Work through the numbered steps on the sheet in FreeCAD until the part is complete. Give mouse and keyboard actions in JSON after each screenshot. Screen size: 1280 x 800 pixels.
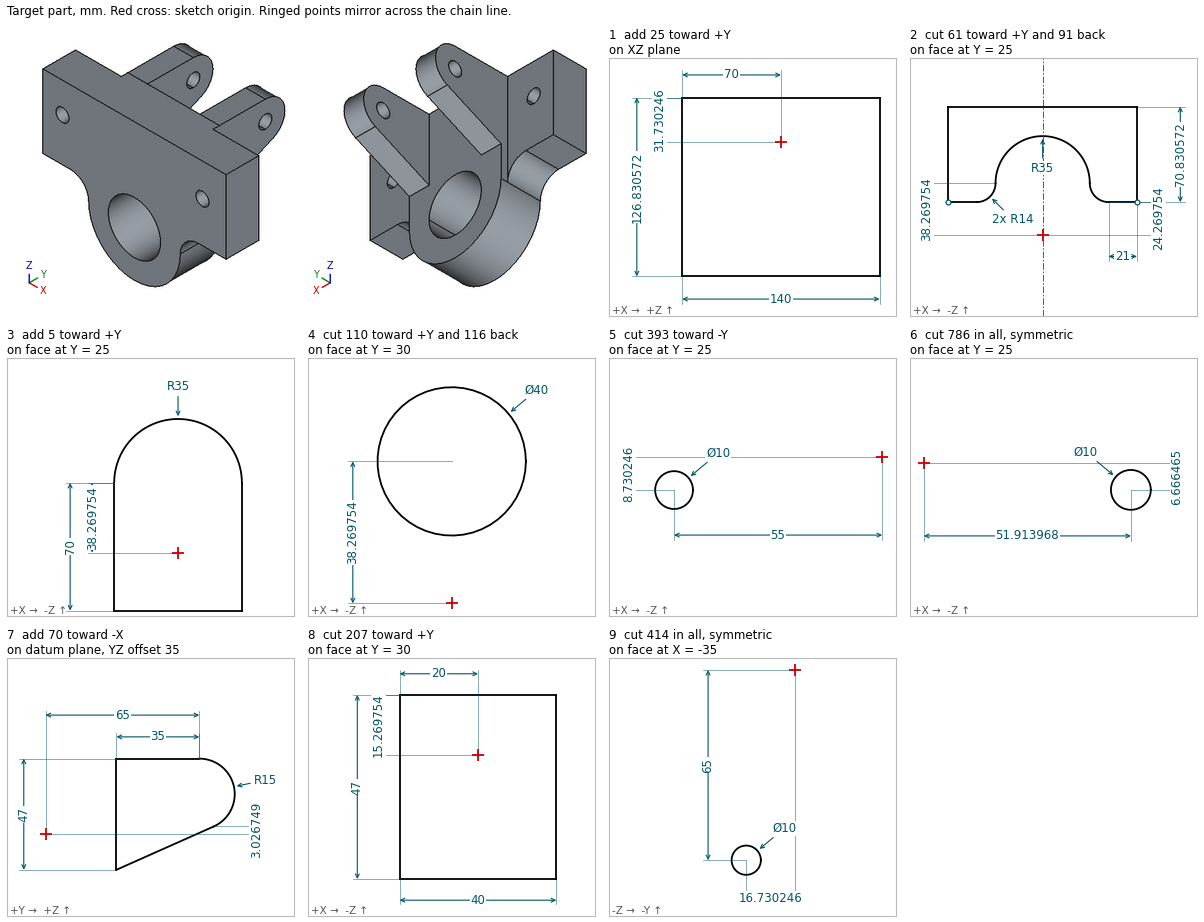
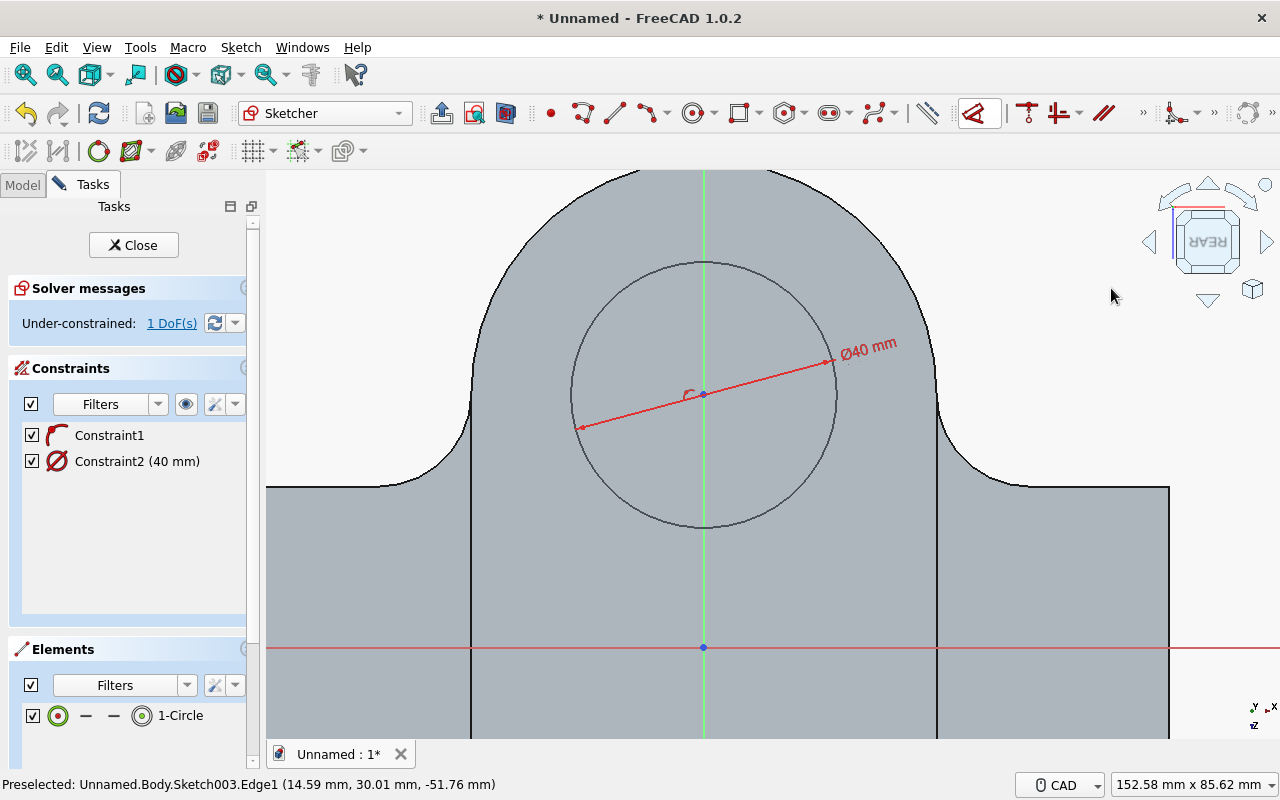
{"action": "left_click", "coordinate": [704, 395]}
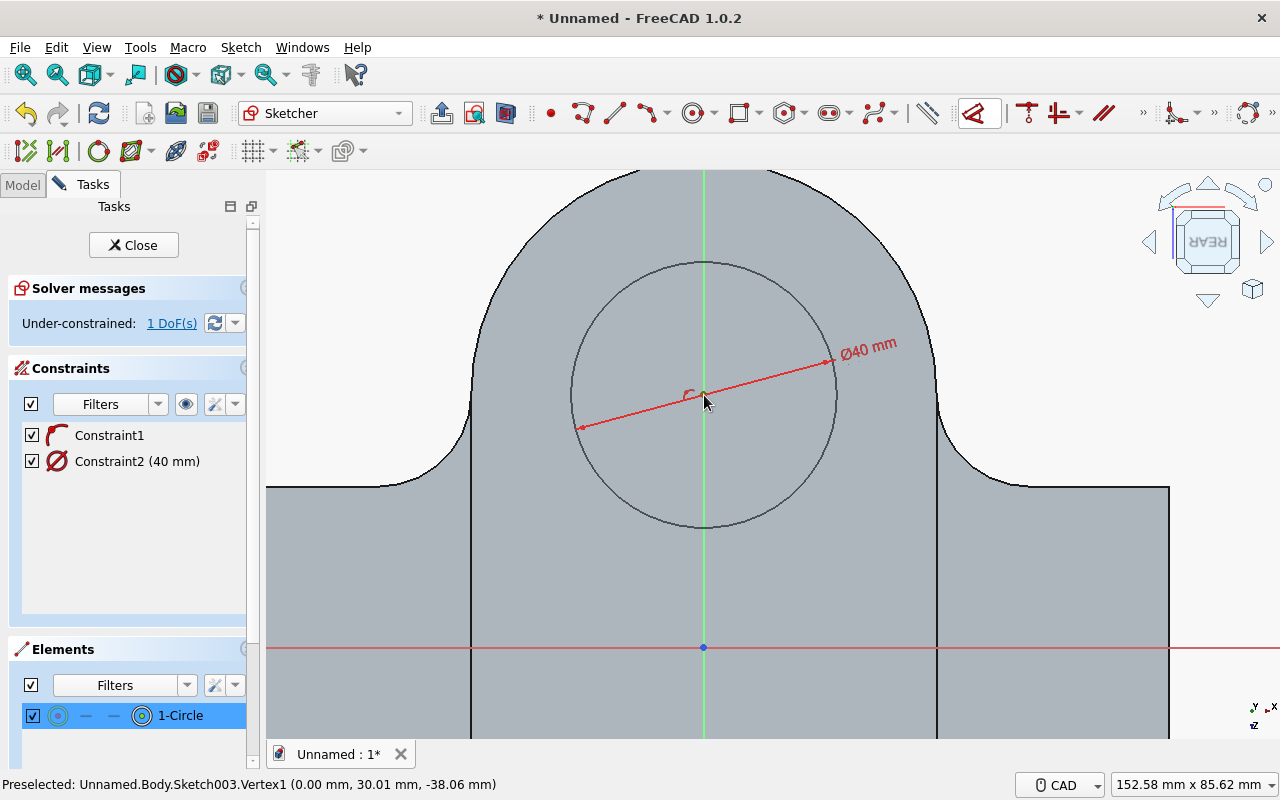
{"action": "key", "text": "i"}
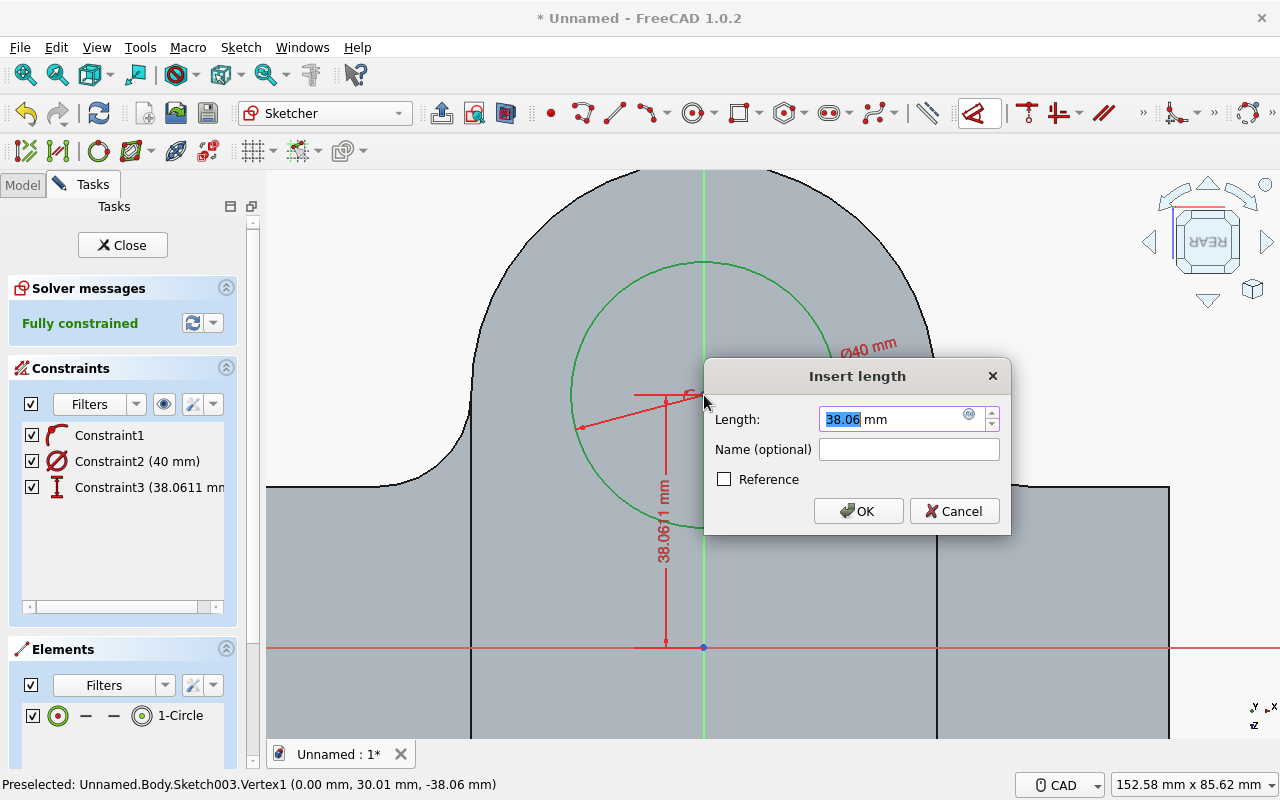
{"action": "type", "text": "38.269754"}
{"action": "key", "text": "Return"}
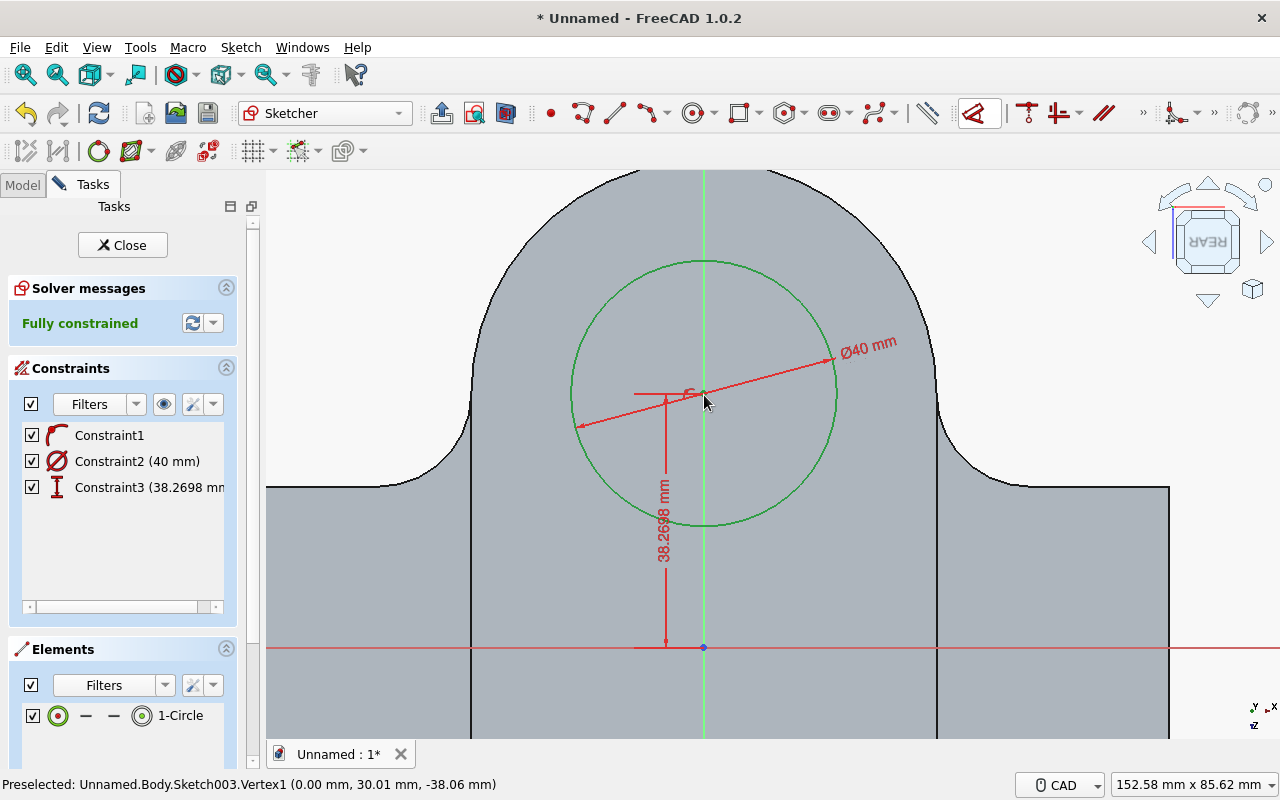
{"action": "left_click", "coordinate": [123, 245]}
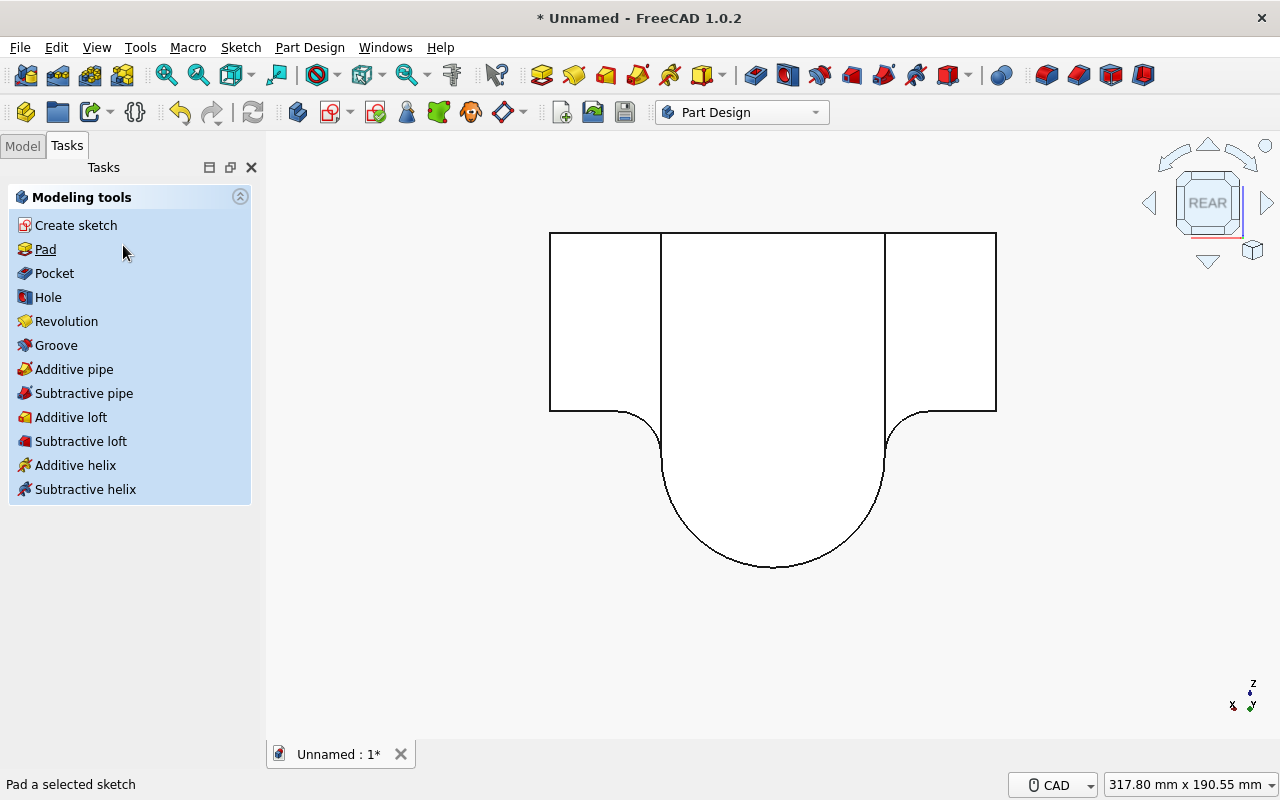
{"action": "left_click", "coordinate": [756, 76]}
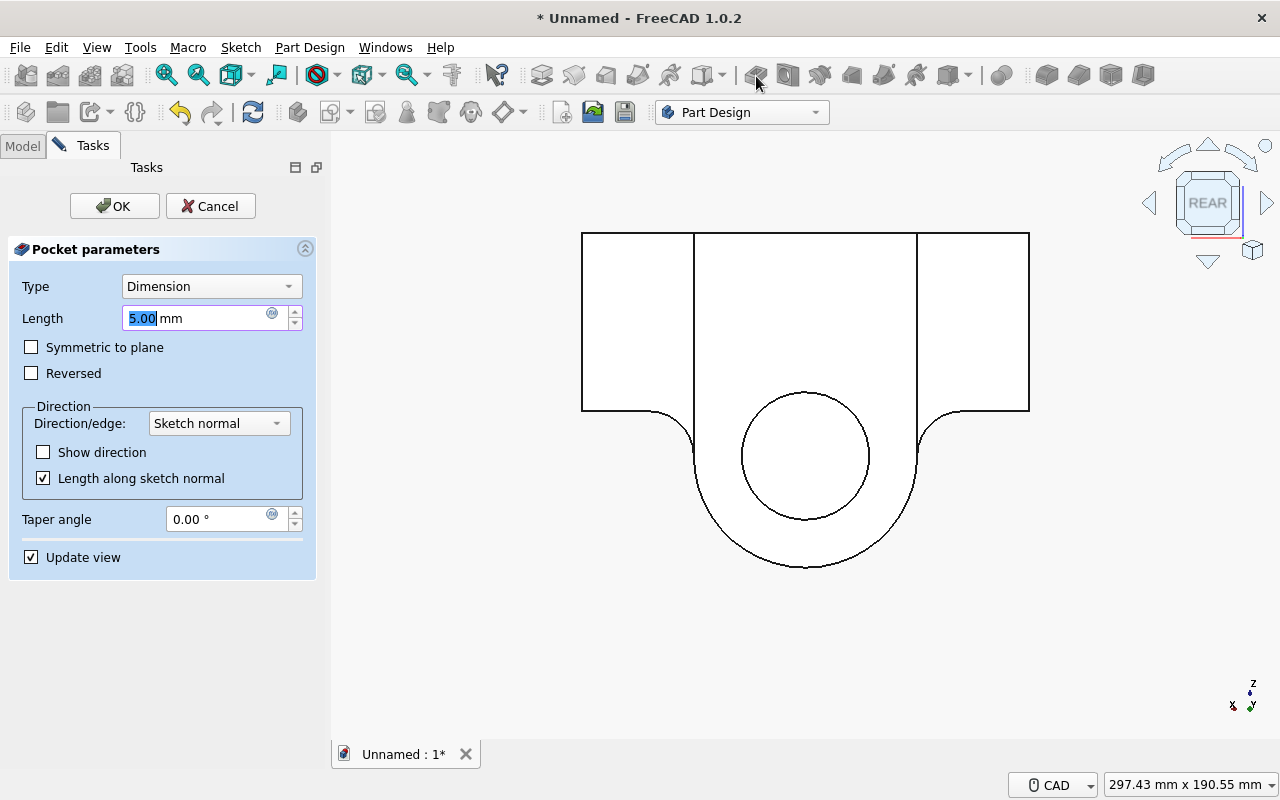
{"action": "left_click", "coordinate": [212, 286]}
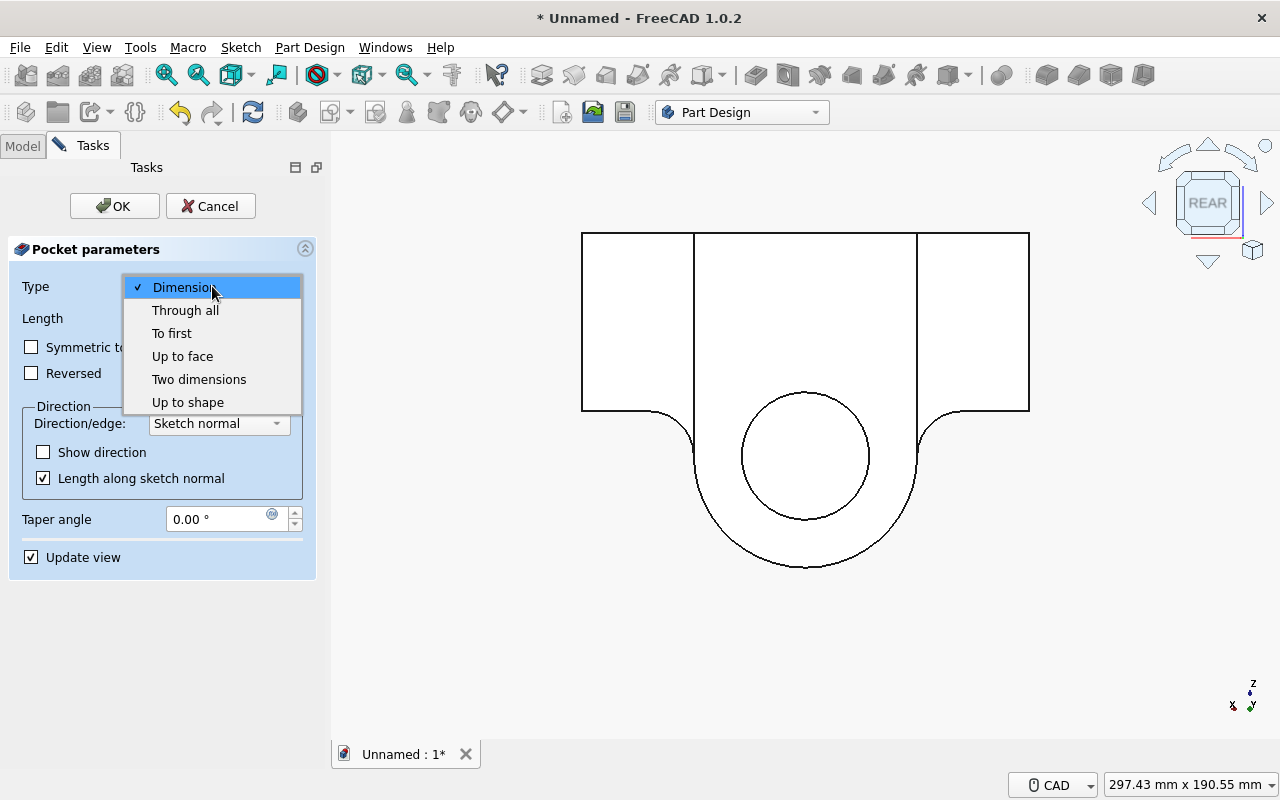
{"action": "left_click", "coordinate": [212, 380]}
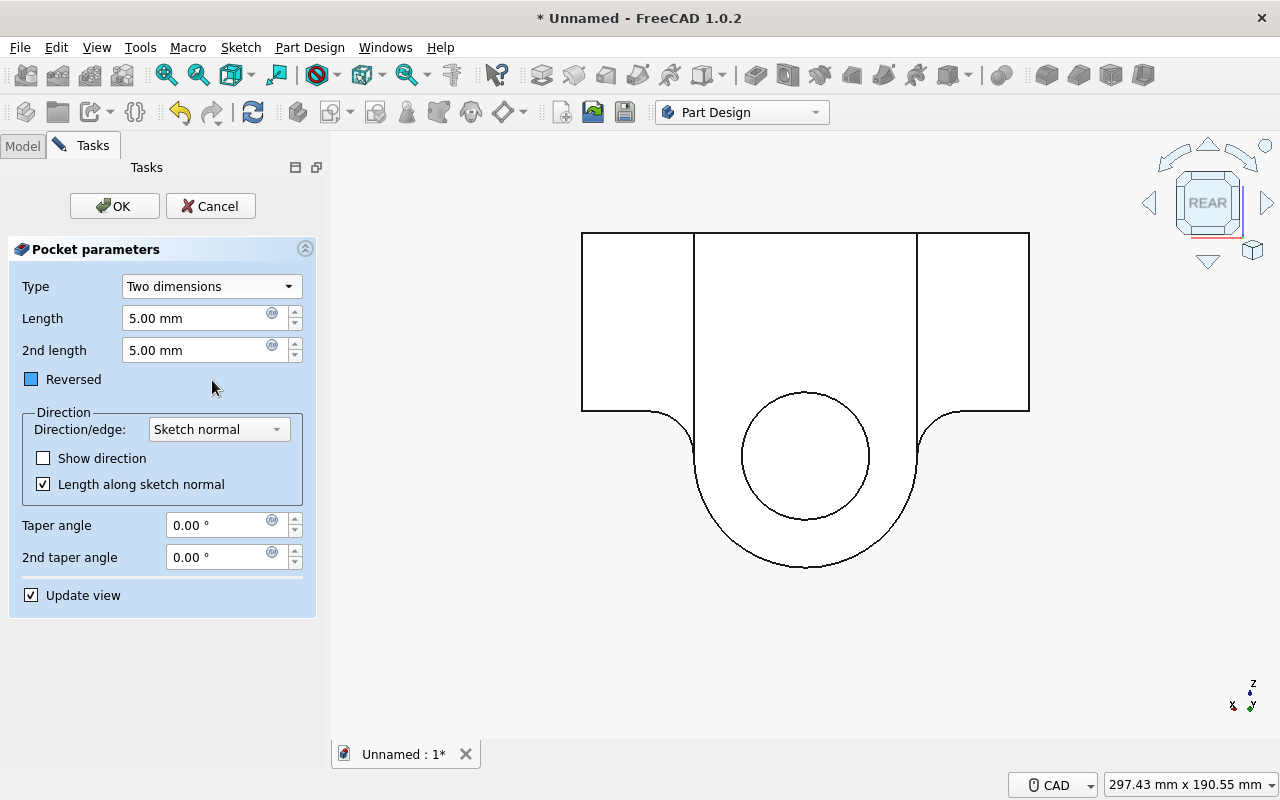
{"action": "triple_click", "coordinate": [204, 318]}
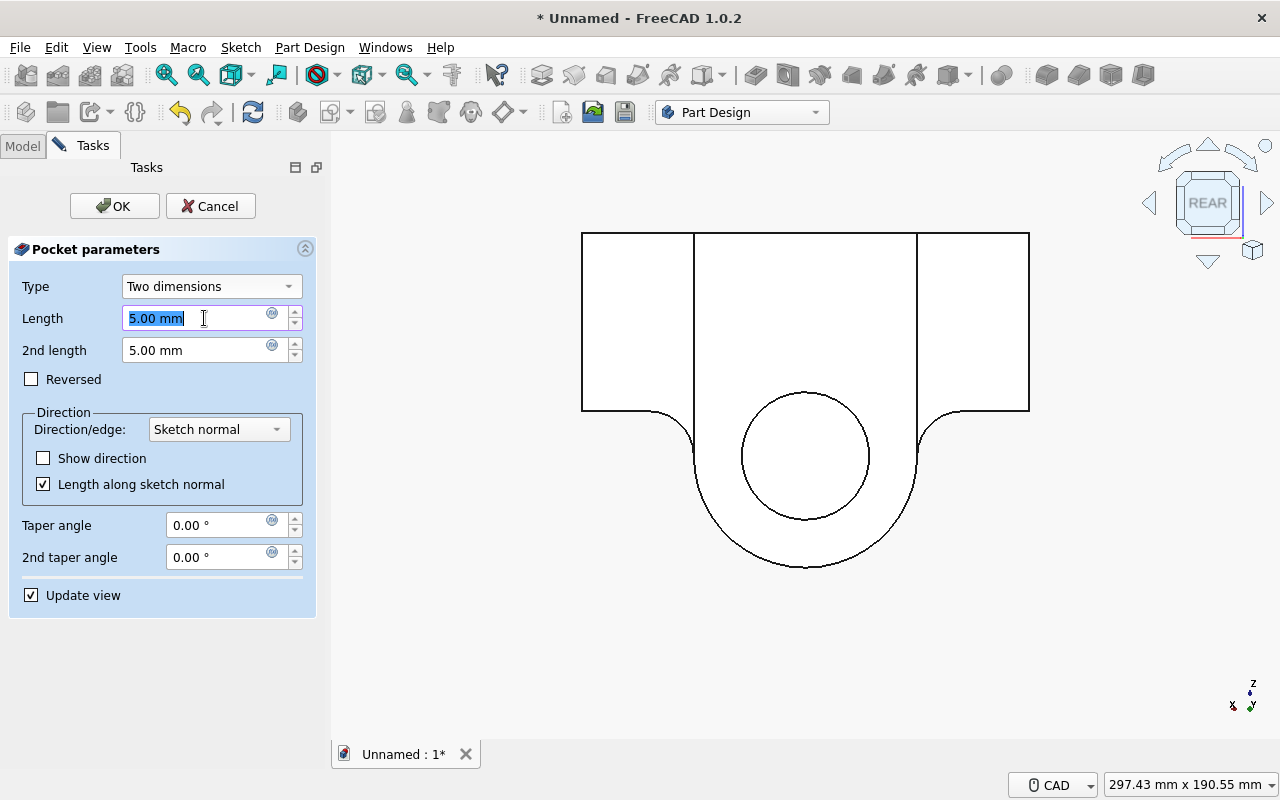
{"action": "type", "text": "110"}
{"action": "key", "text": "Tab"}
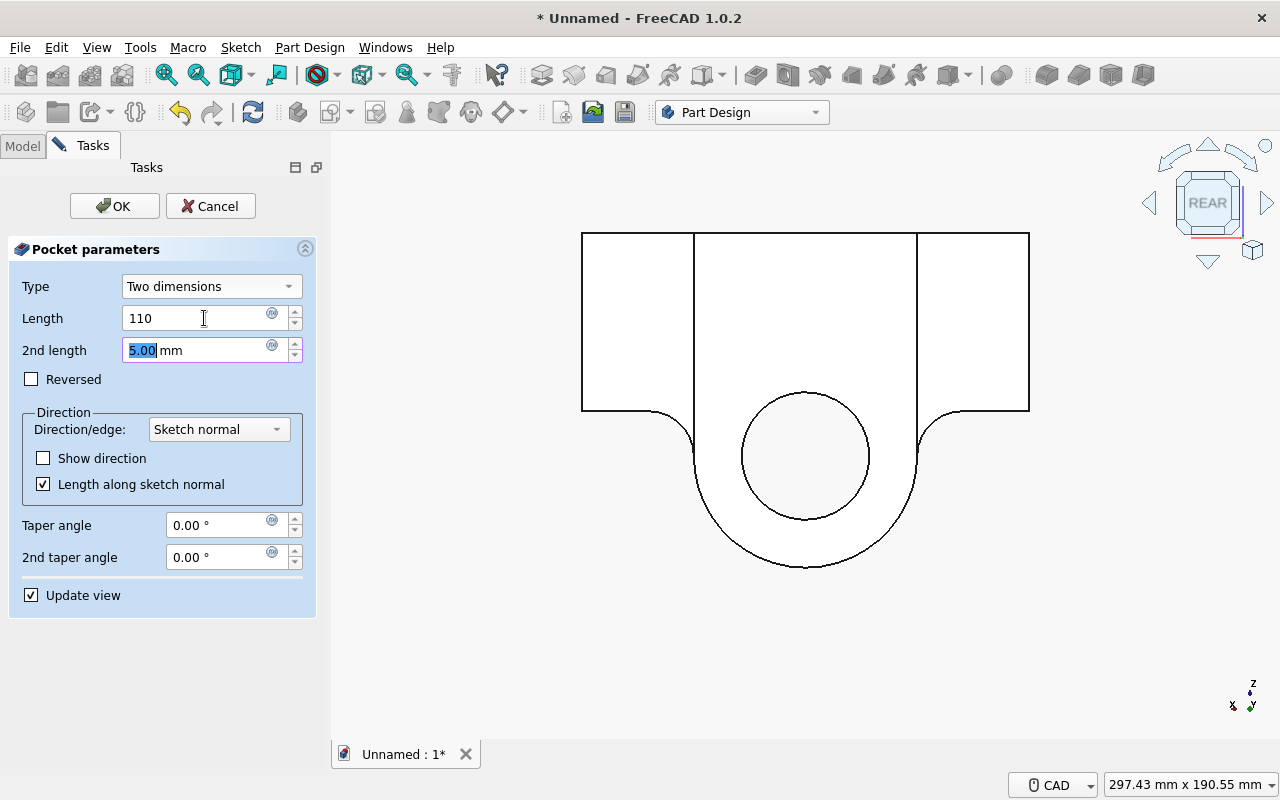
{"action": "type", "text": "116"}
{"action": "key", "text": "Tab"}